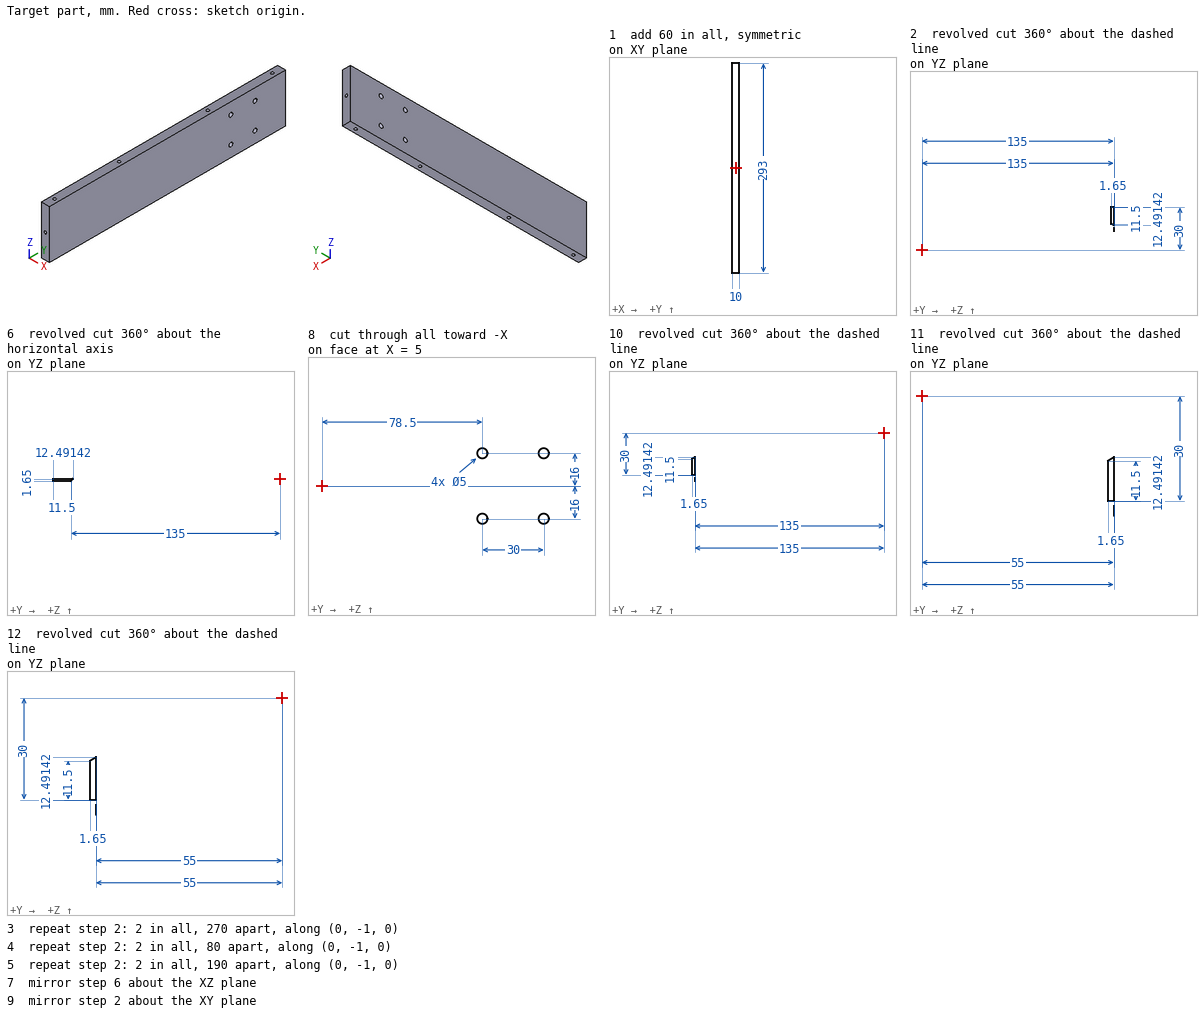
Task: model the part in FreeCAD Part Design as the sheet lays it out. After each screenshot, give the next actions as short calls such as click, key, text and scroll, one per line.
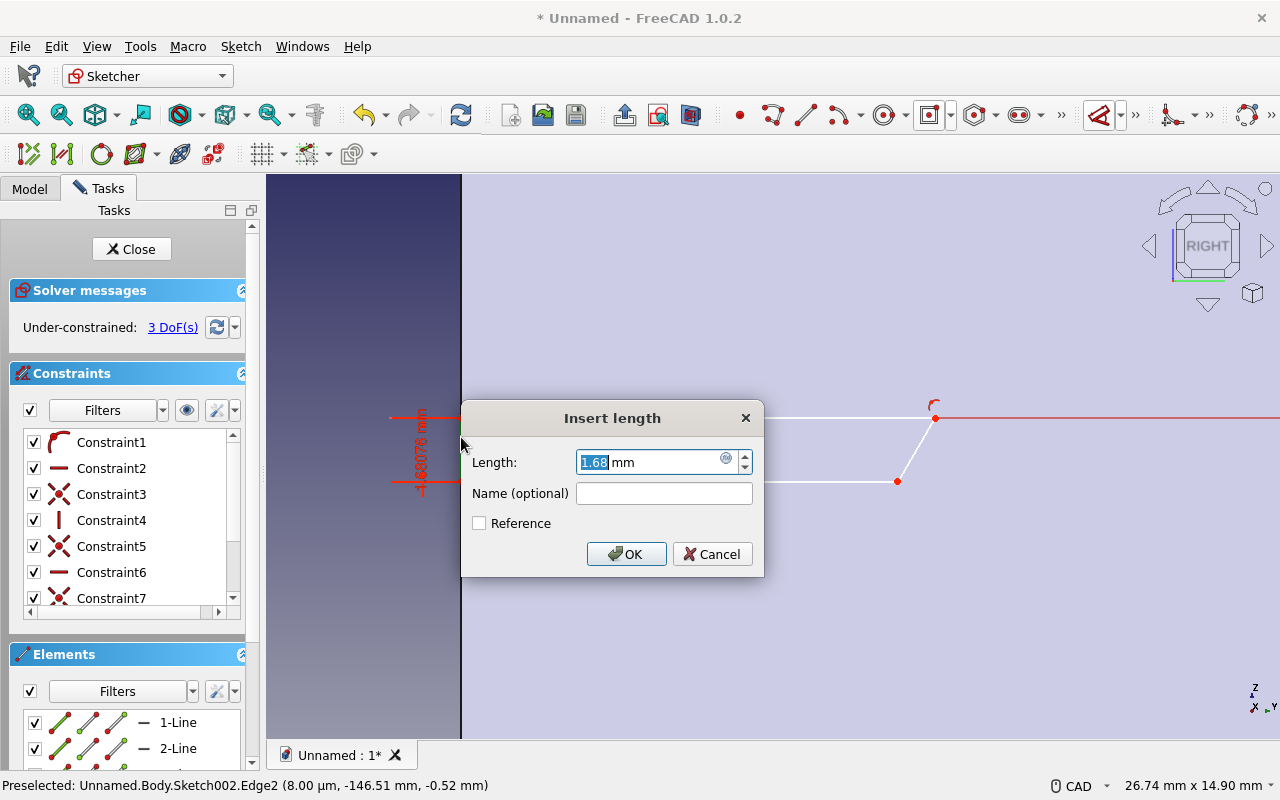
text(1.65)
key(Return)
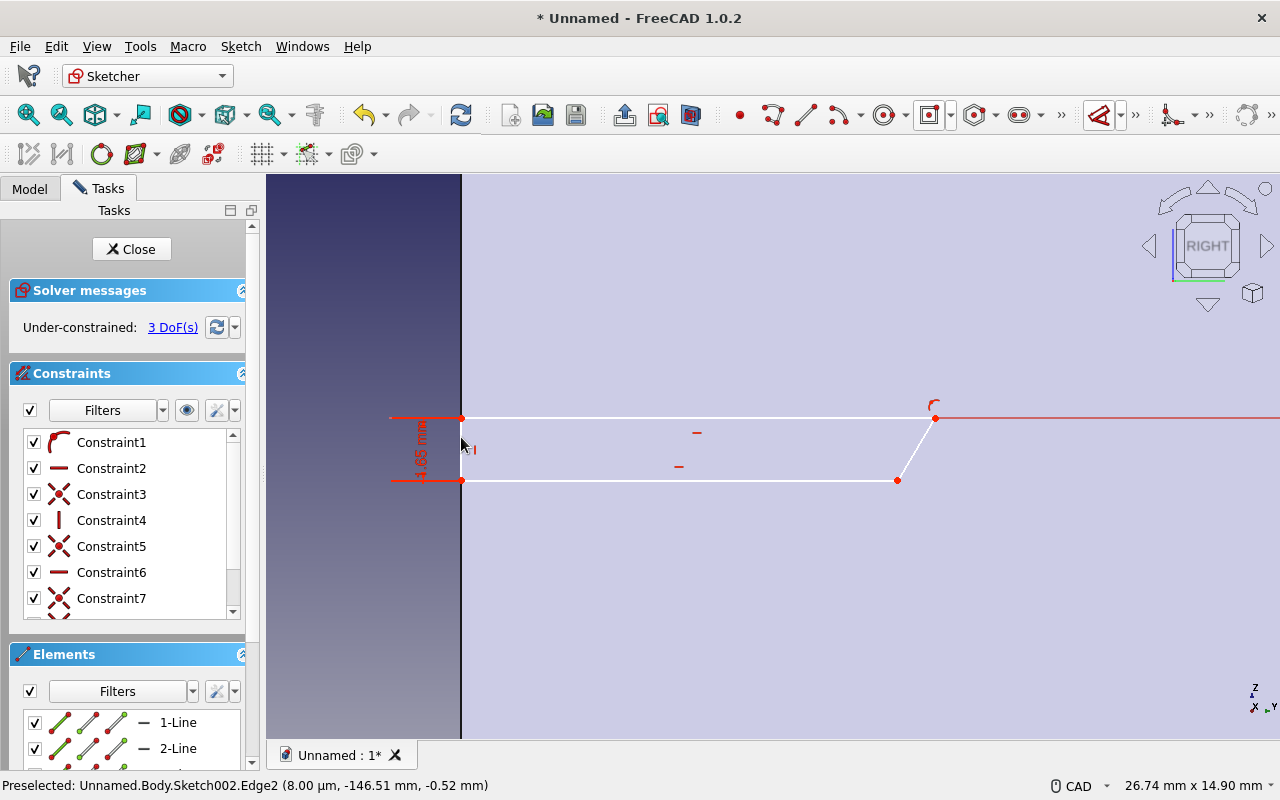
click(592, 481)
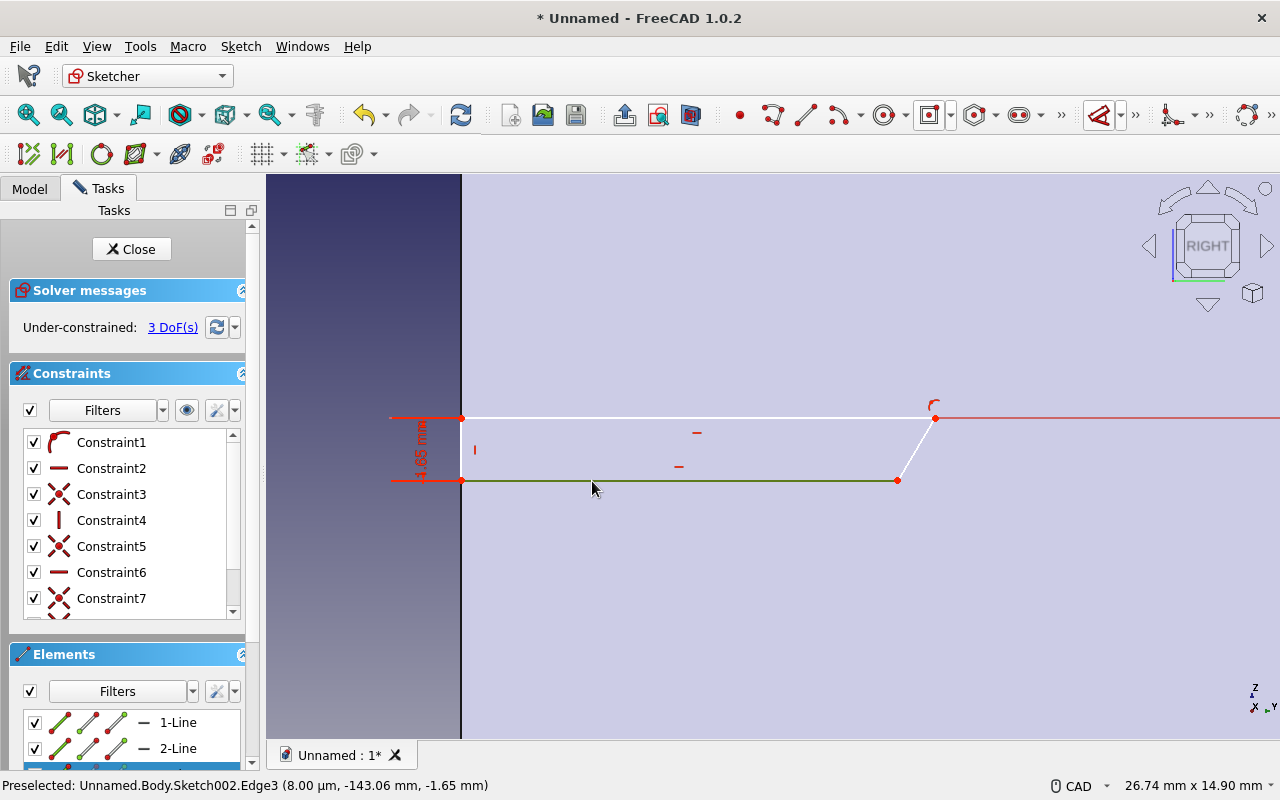
click(1120, 116)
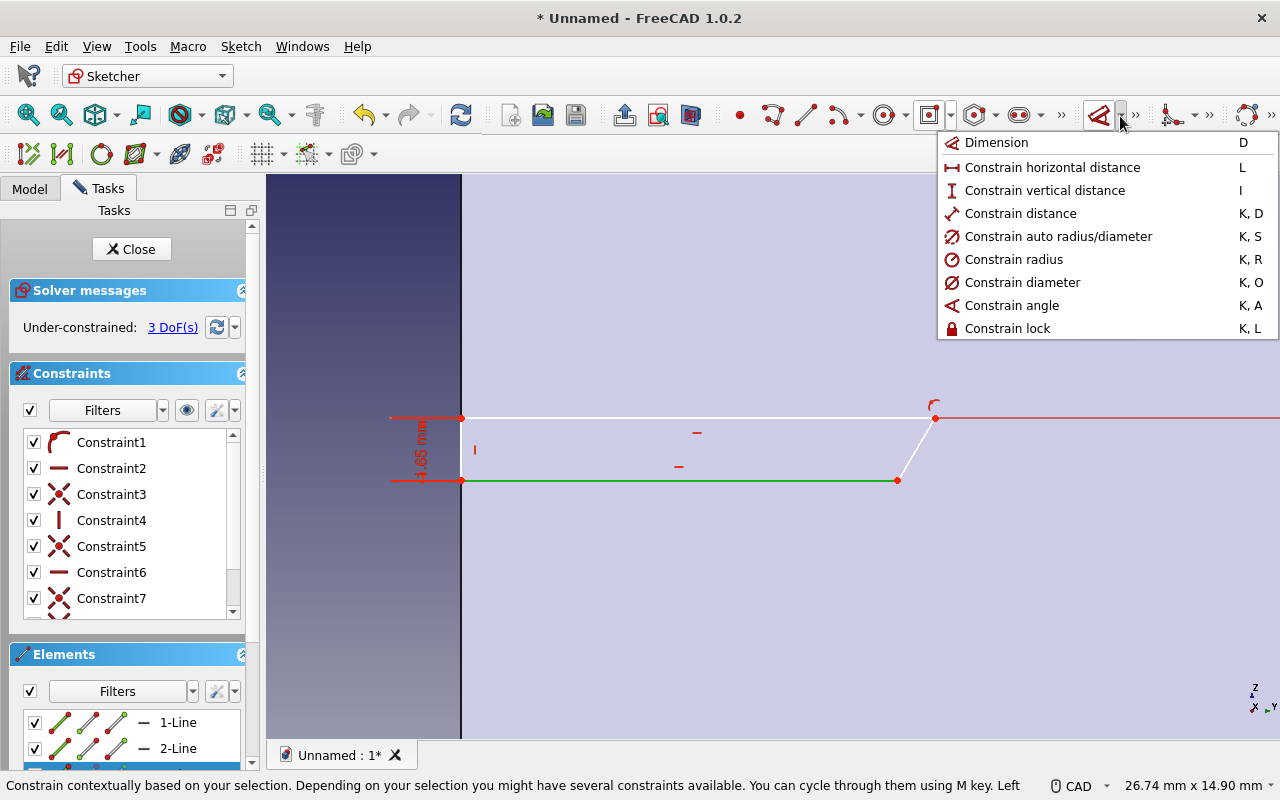
click(1108, 168)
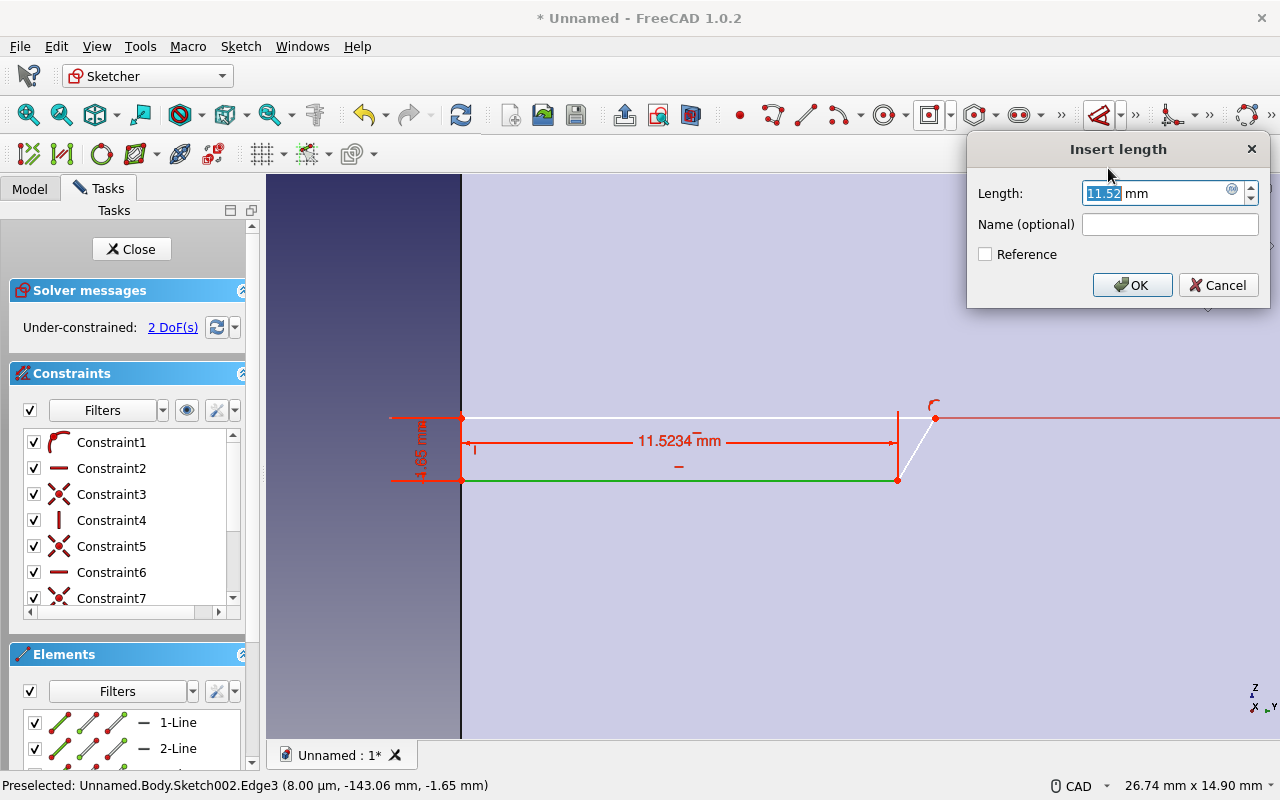
text(11.5)
key(Return)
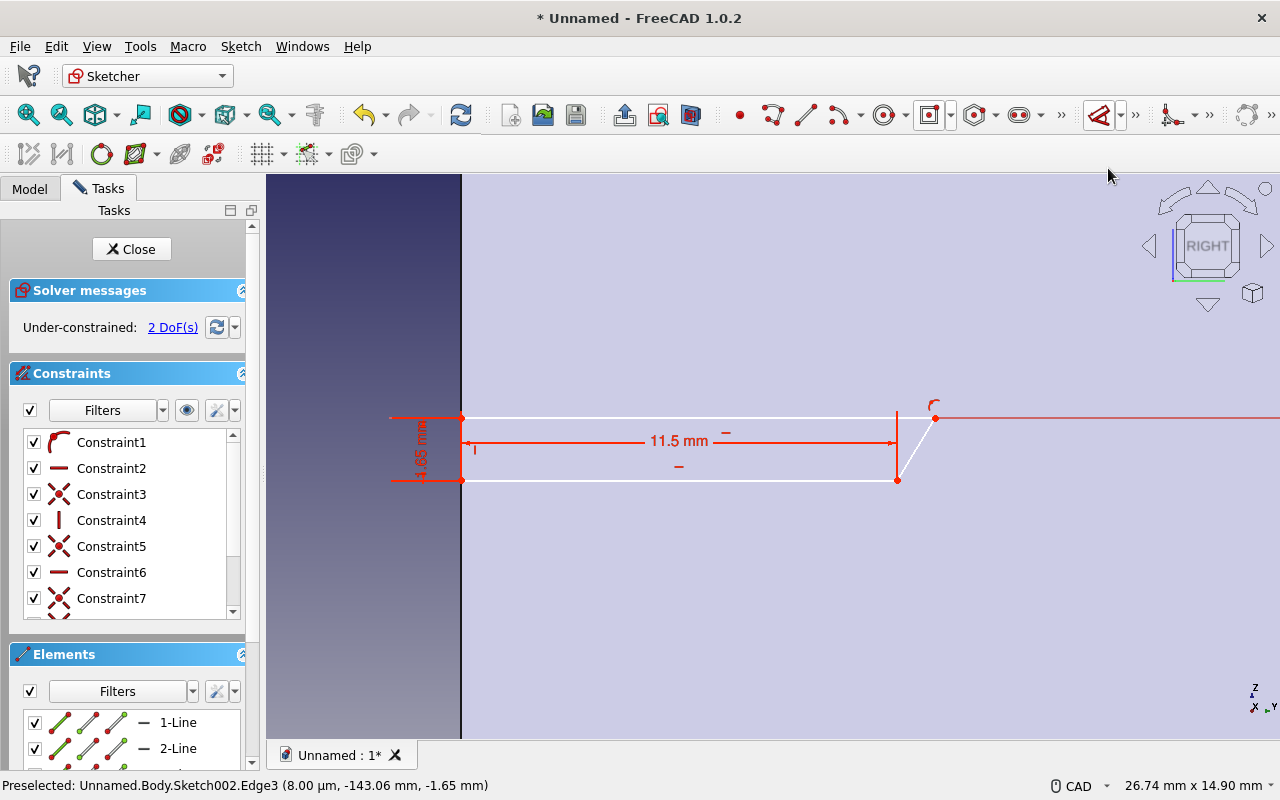
click(897, 481)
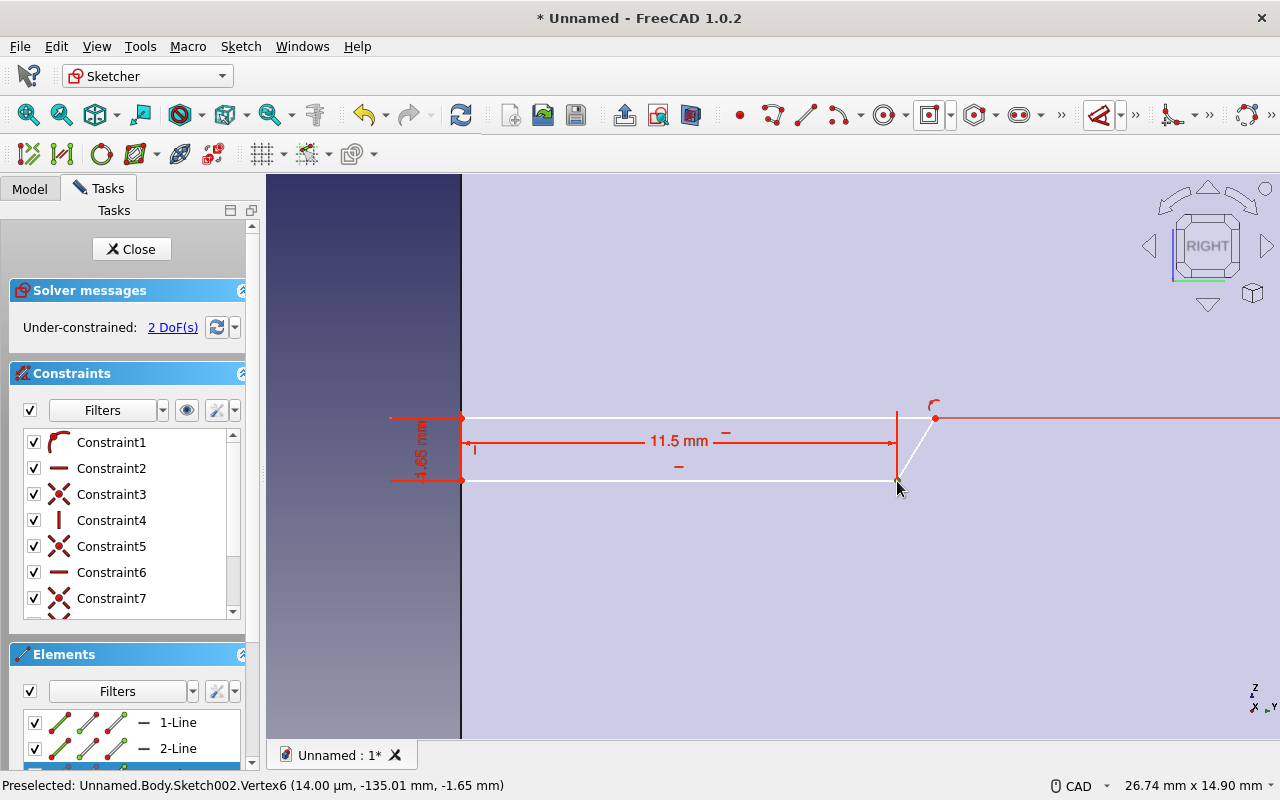
click(1120, 116)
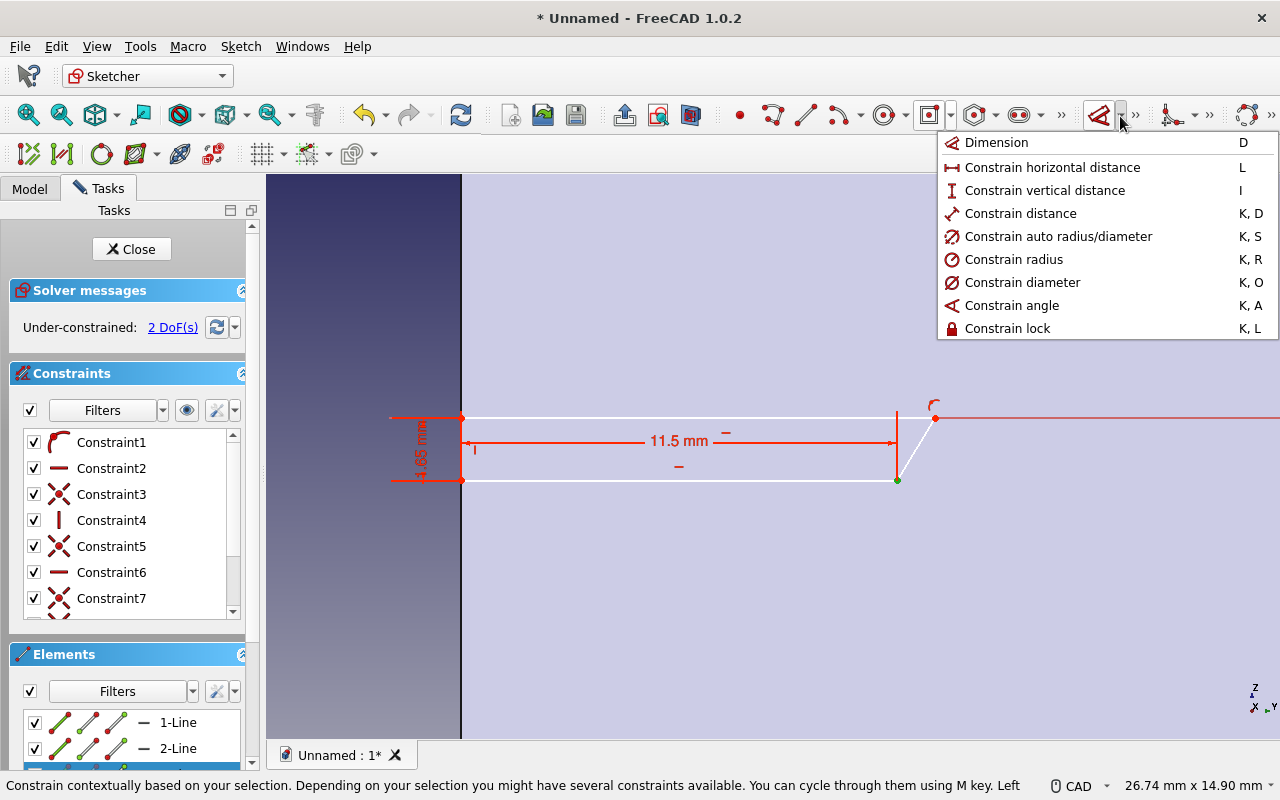
click(1108, 168)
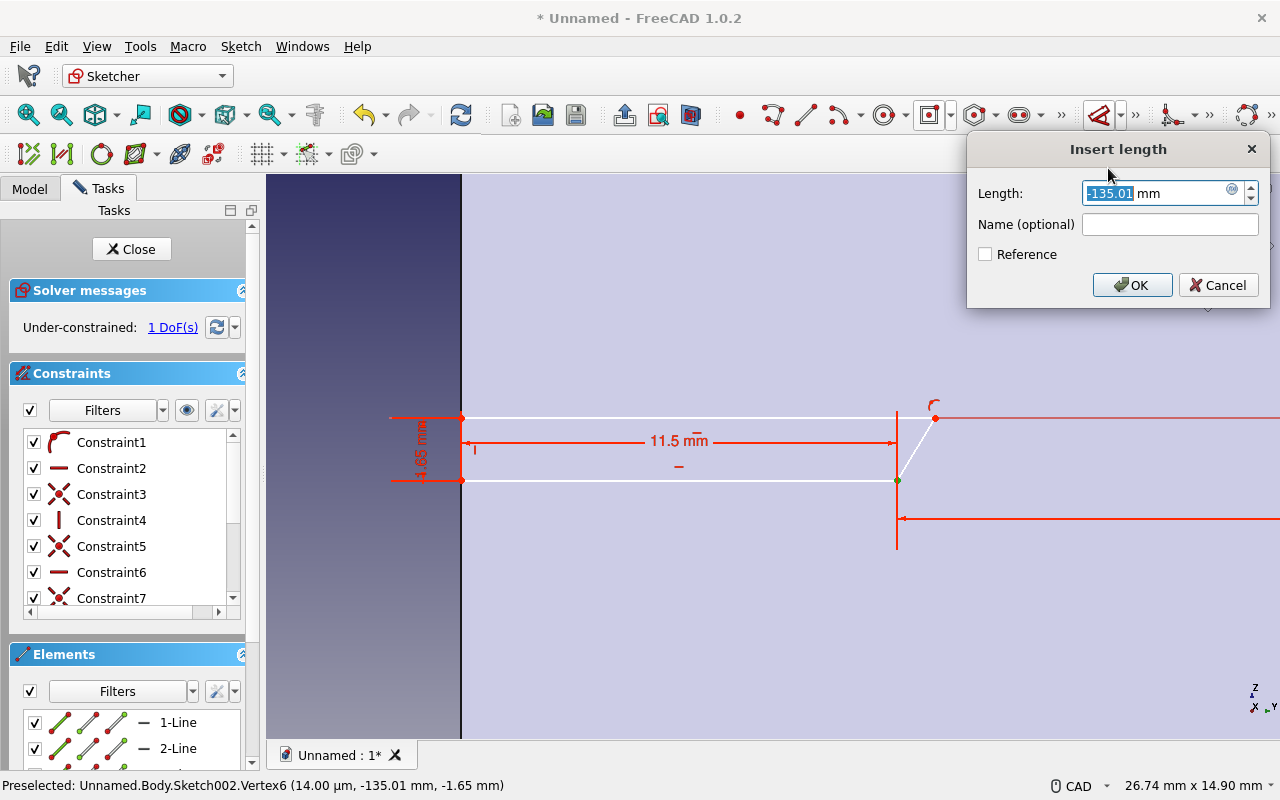
text(-135)
key(Return)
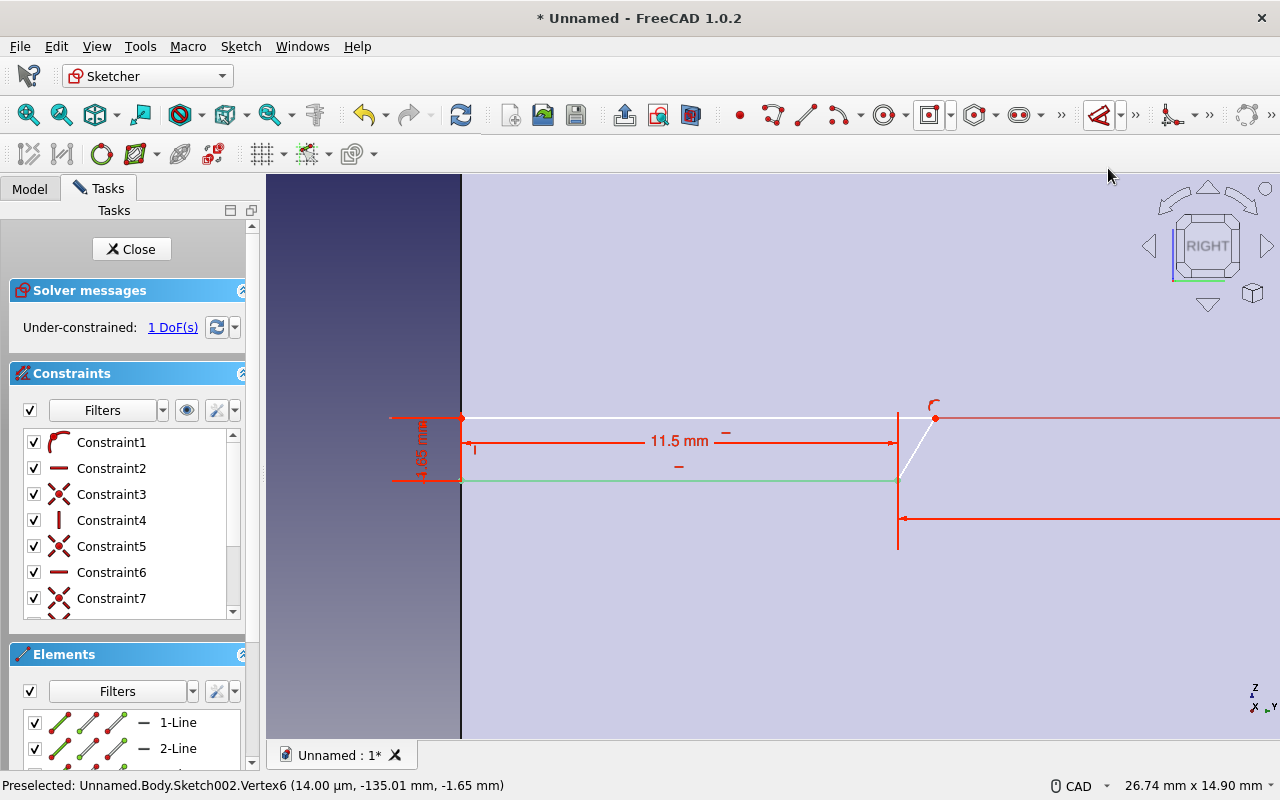
click(793, 418)